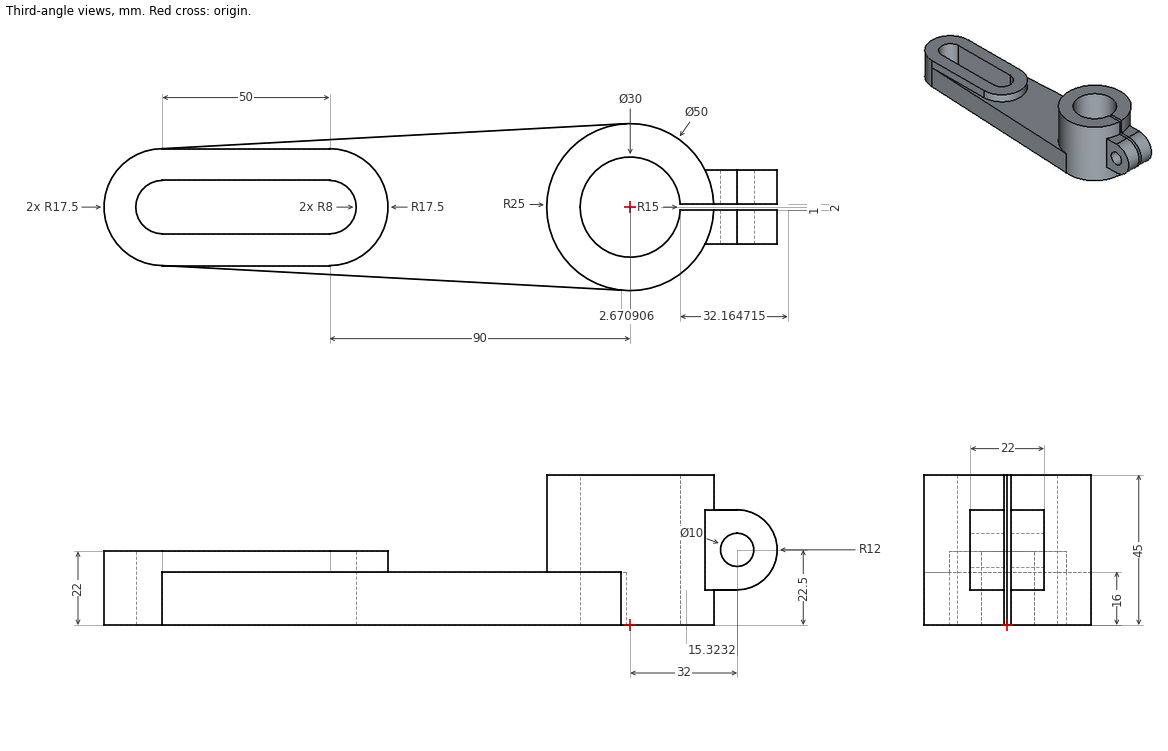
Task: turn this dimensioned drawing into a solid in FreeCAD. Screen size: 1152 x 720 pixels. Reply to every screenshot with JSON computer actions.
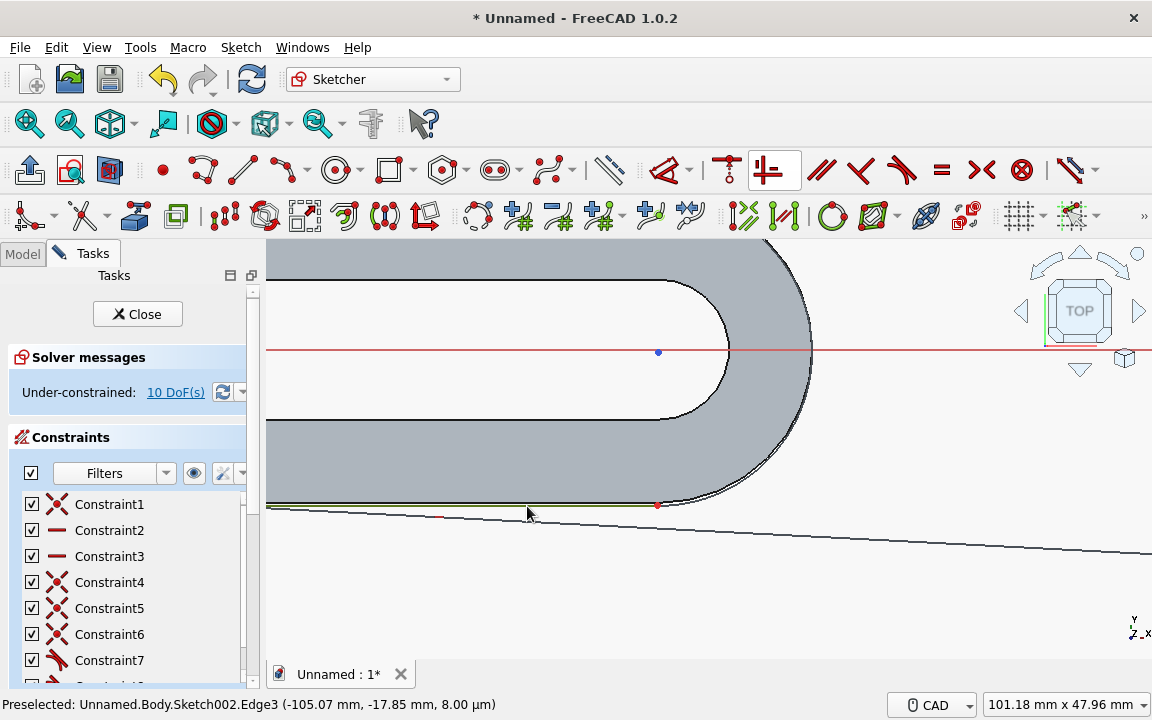
{"action": "left_click", "coordinate": [783, 443]}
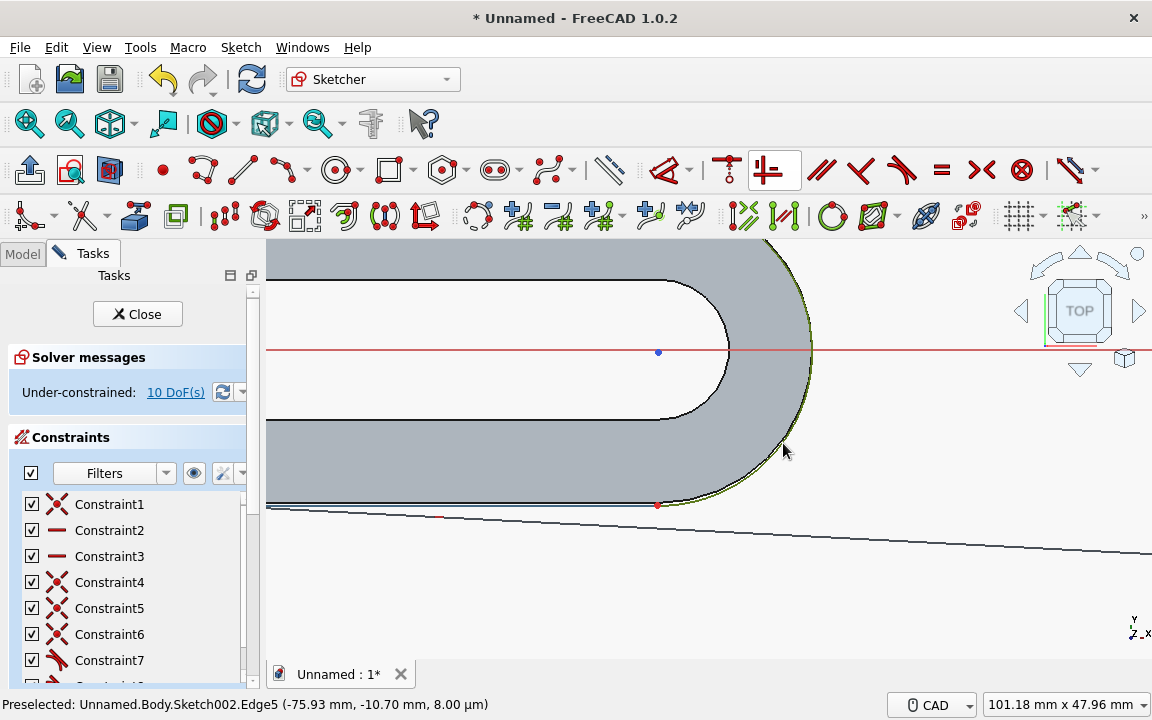
{"action": "key", "text": "t"}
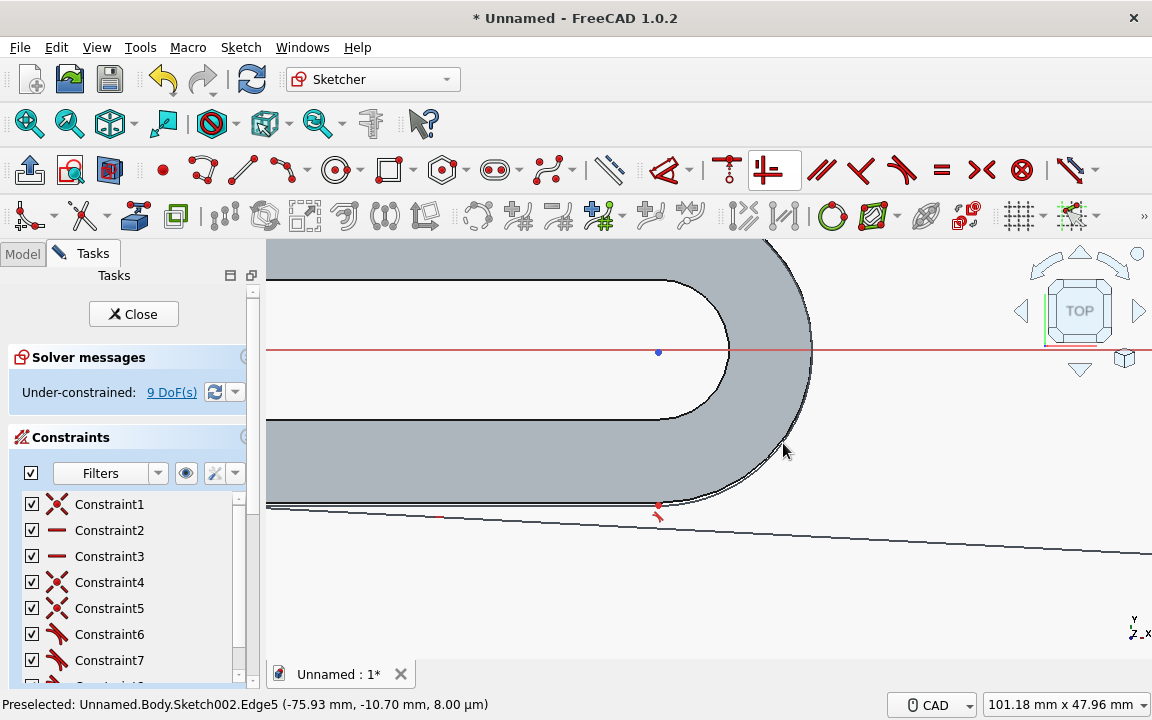
{"action": "scroll", "coordinate": [528, 507], "scroll_direction": "down", "scroll_amount": 5}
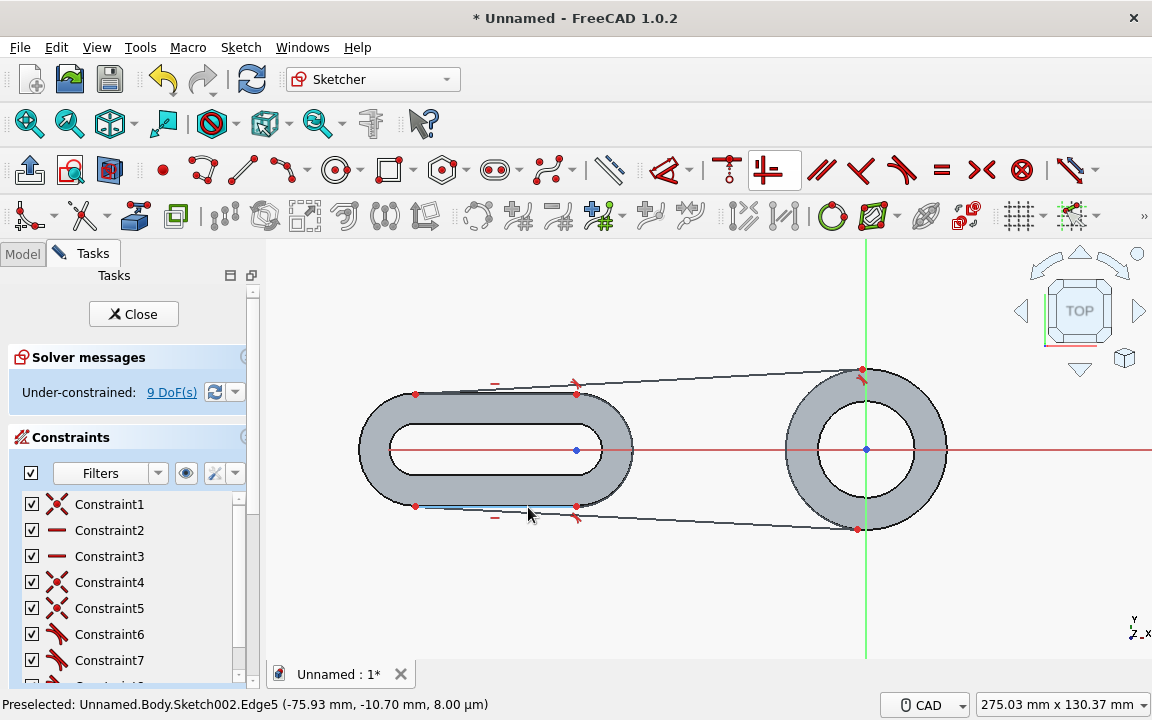
{"action": "left_click_drag", "start_coordinate": [856, 440], "coordinate": [876, 460]}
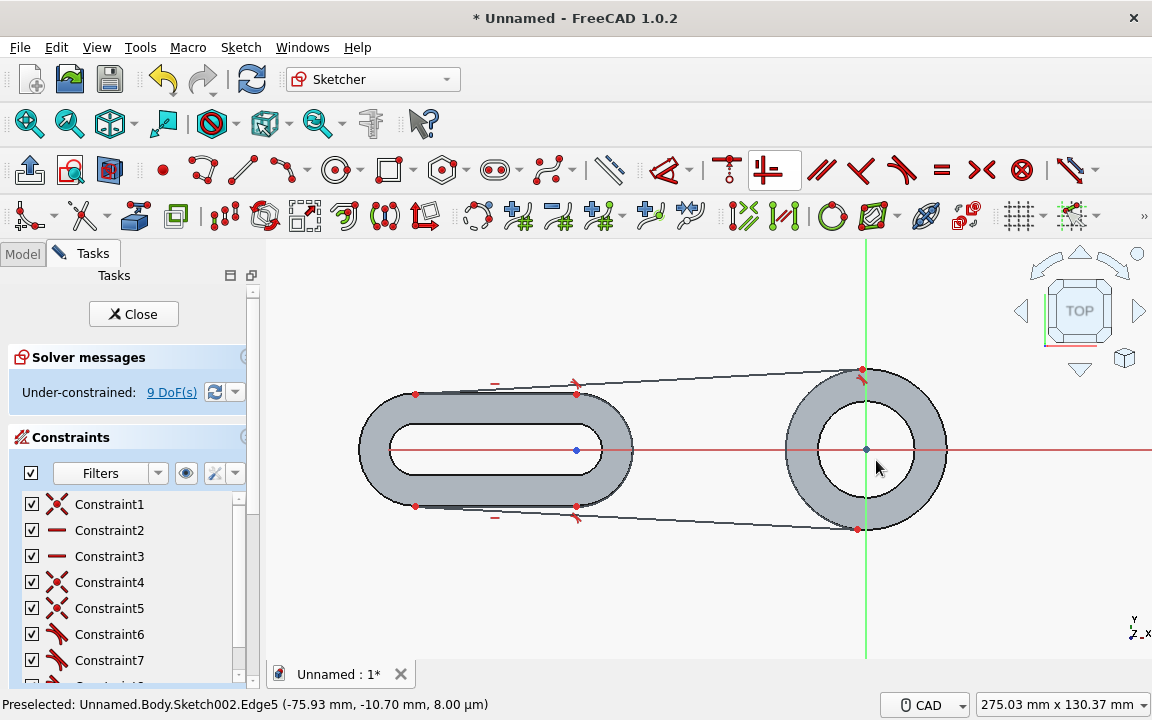
{"action": "left_click", "coordinate": [728, 170]}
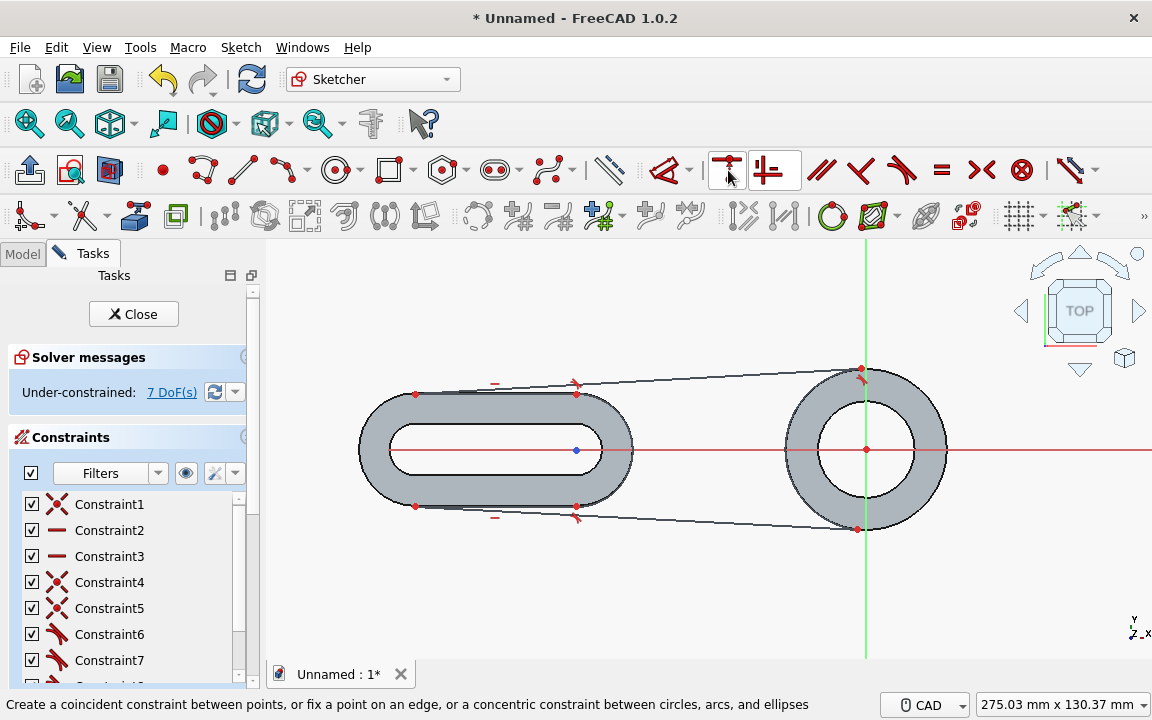
{"action": "left_click", "coordinate": [576, 451]}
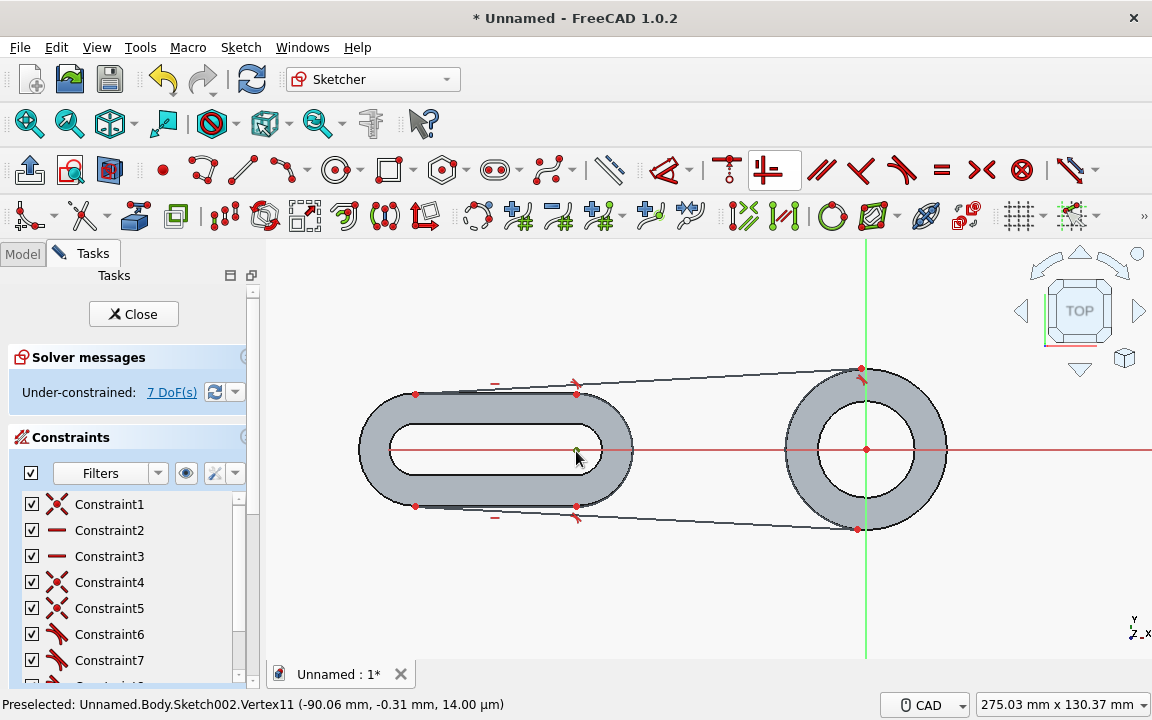
{"action": "left_click", "coordinate": [393, 450]}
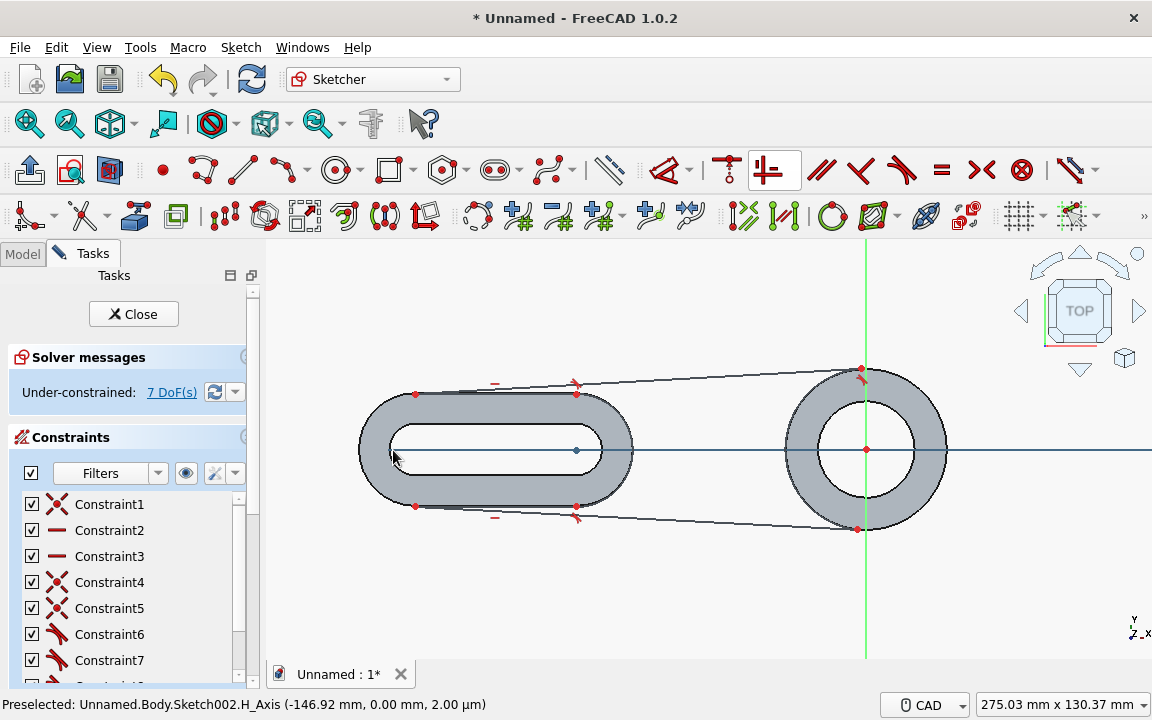
{"action": "key", "text": "c"}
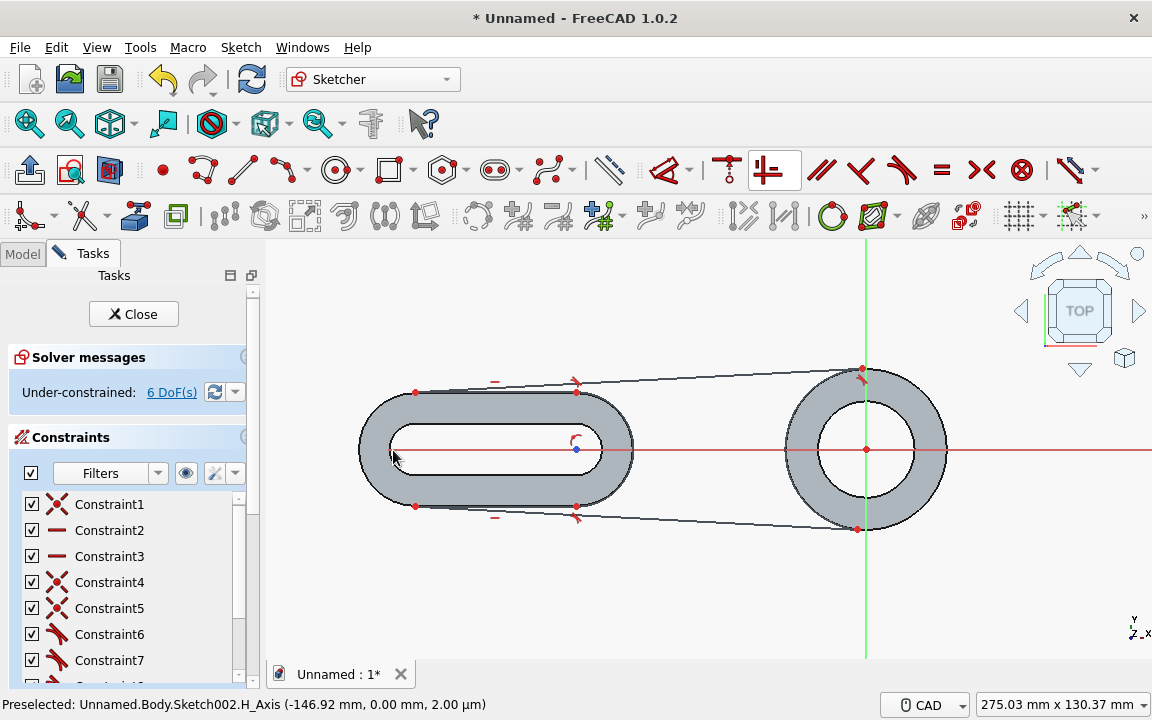
{"action": "left_click", "coordinate": [664, 170]}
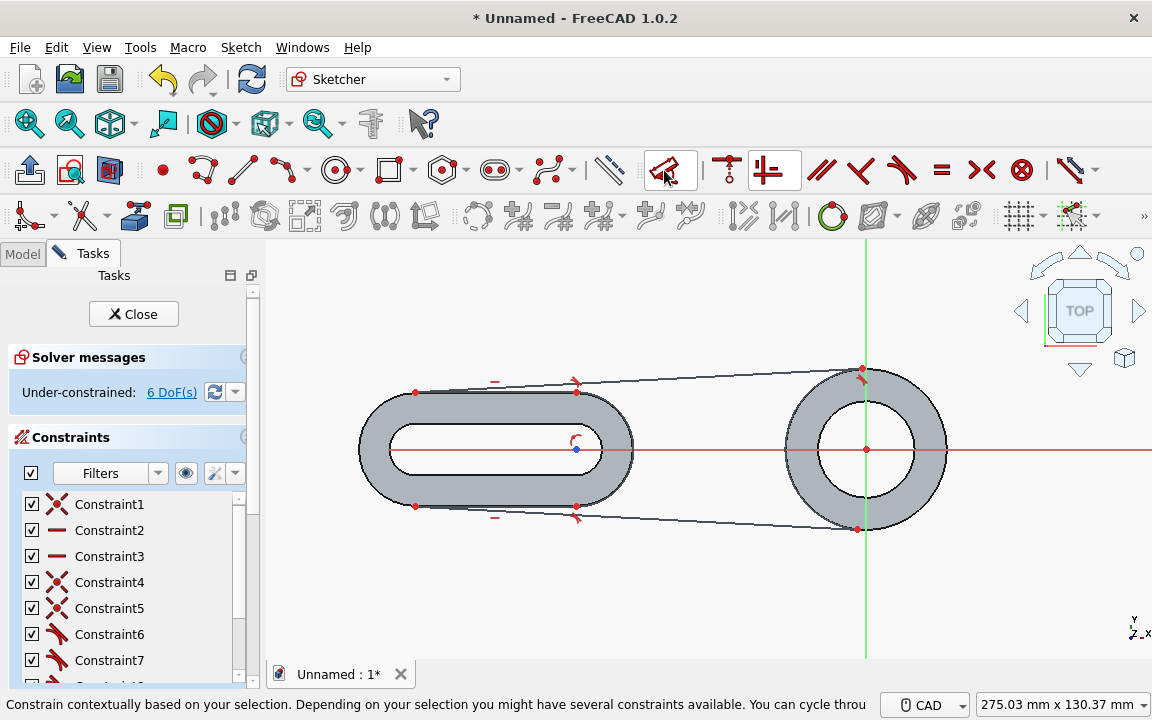
{"action": "left_click", "coordinate": [622, 483]}
{"action": "left_click", "coordinate": [648, 502]}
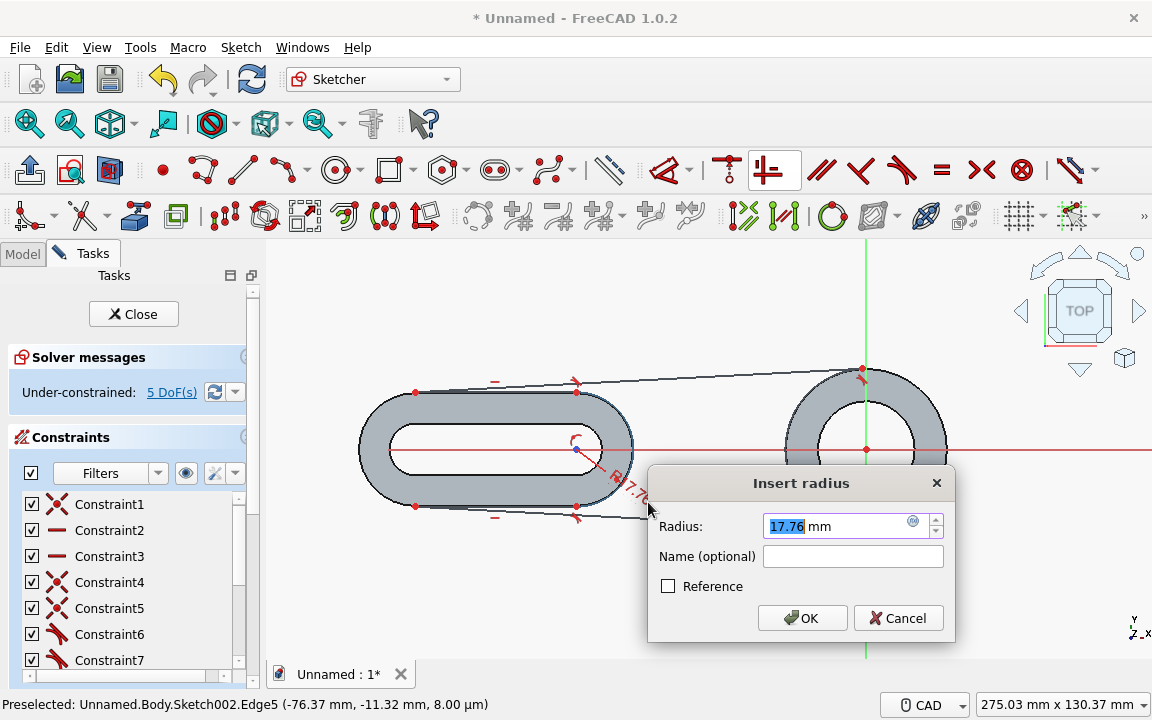
{"action": "type", "text": "17.5"}
{"action": "key", "text": "Return"}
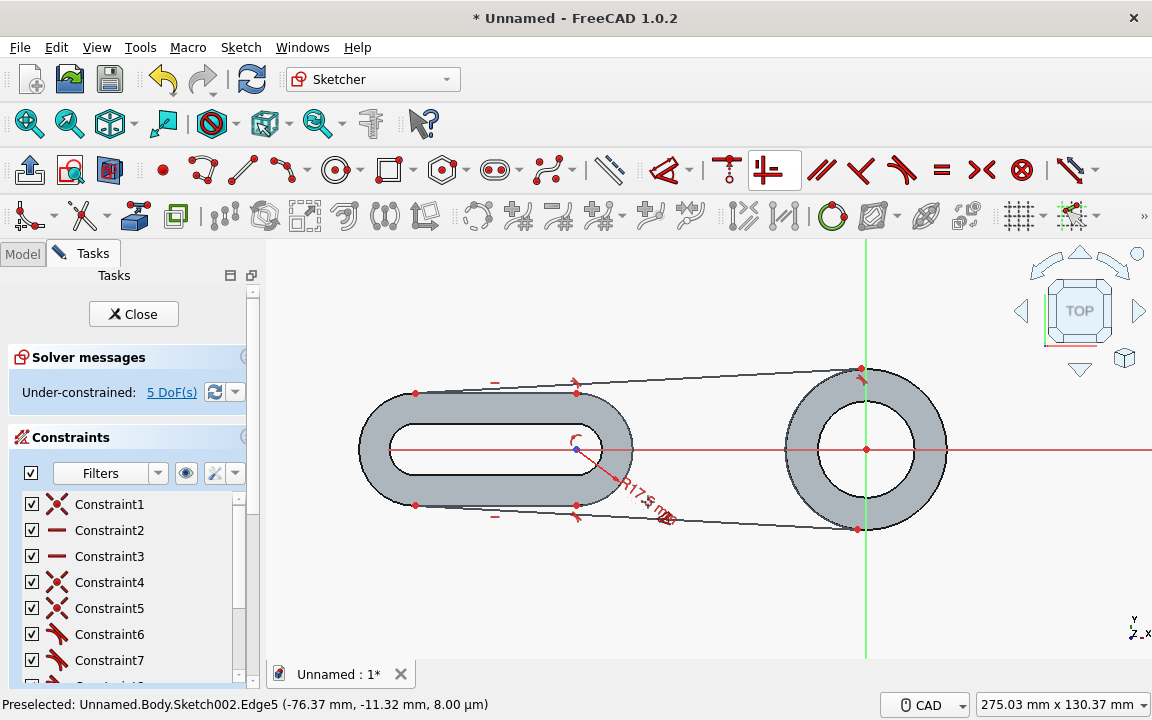
{"action": "left_click", "coordinate": [801, 402]}
{"action": "left_click", "coordinate": [818, 348]}